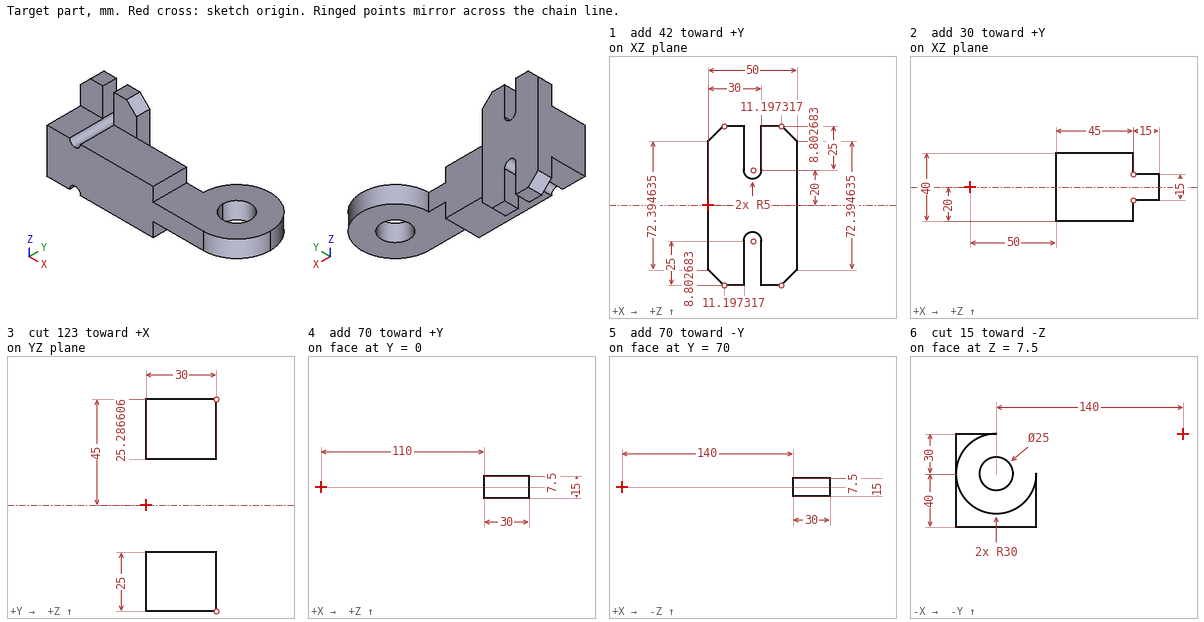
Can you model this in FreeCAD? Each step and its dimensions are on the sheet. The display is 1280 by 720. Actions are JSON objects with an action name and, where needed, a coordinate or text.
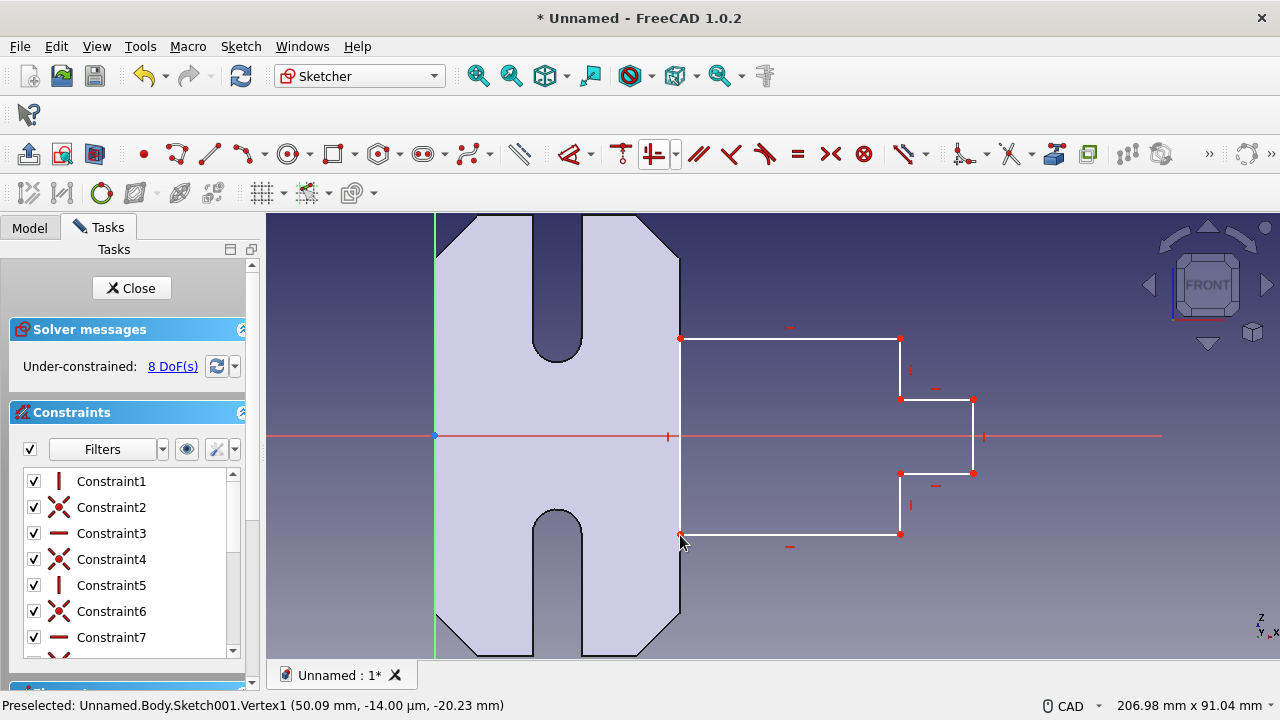
{"action": "left_click", "coordinate": [900, 400]}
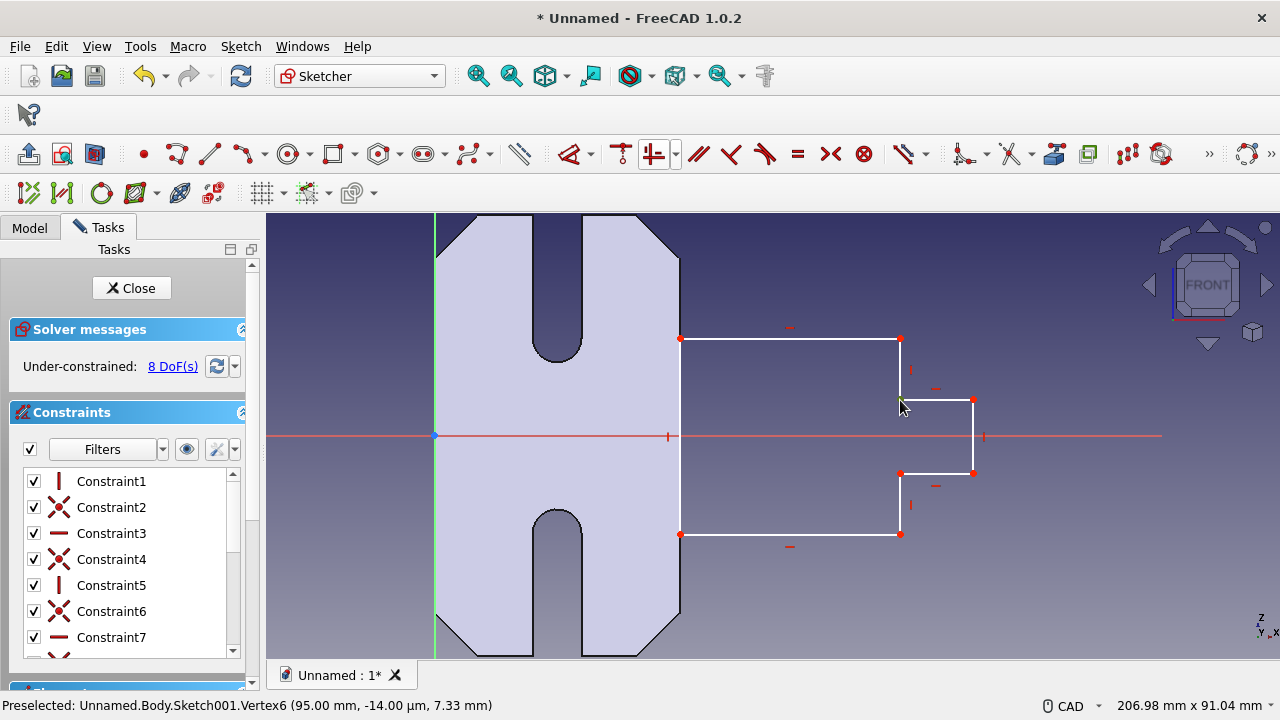
{"action": "left_click", "coordinate": [900, 474]}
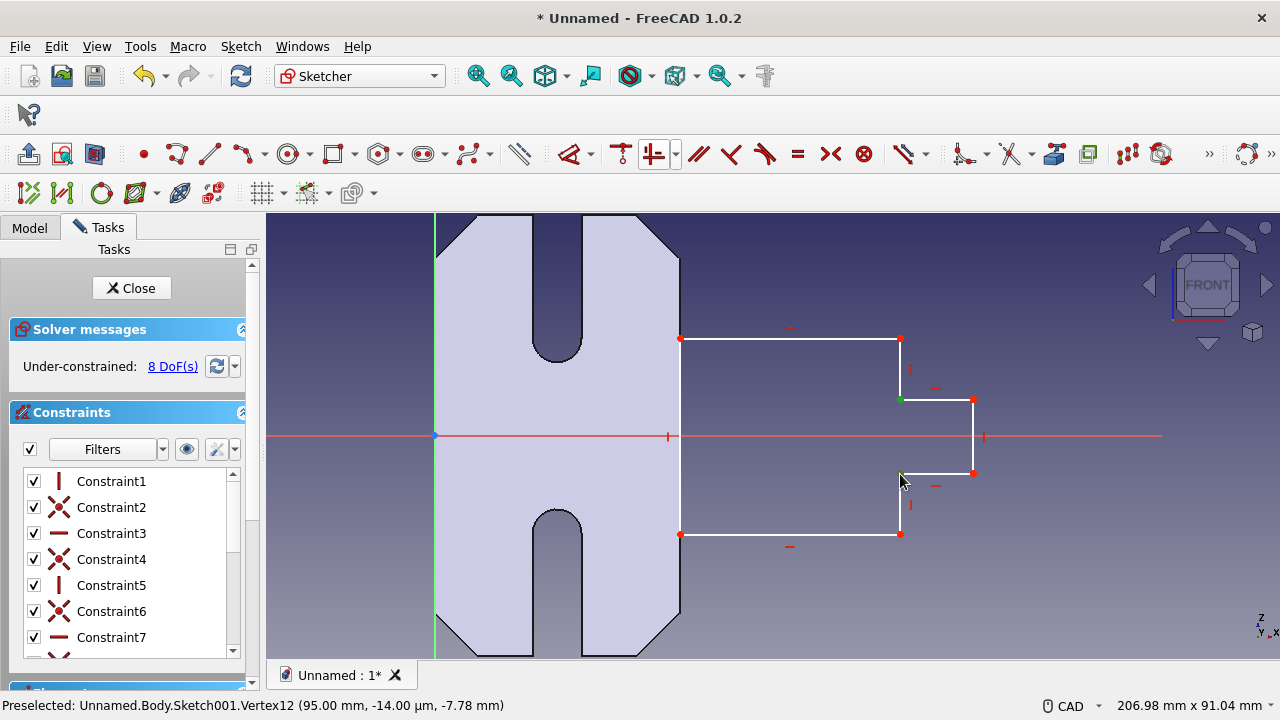
{"action": "left_click", "coordinate": [353, 436]}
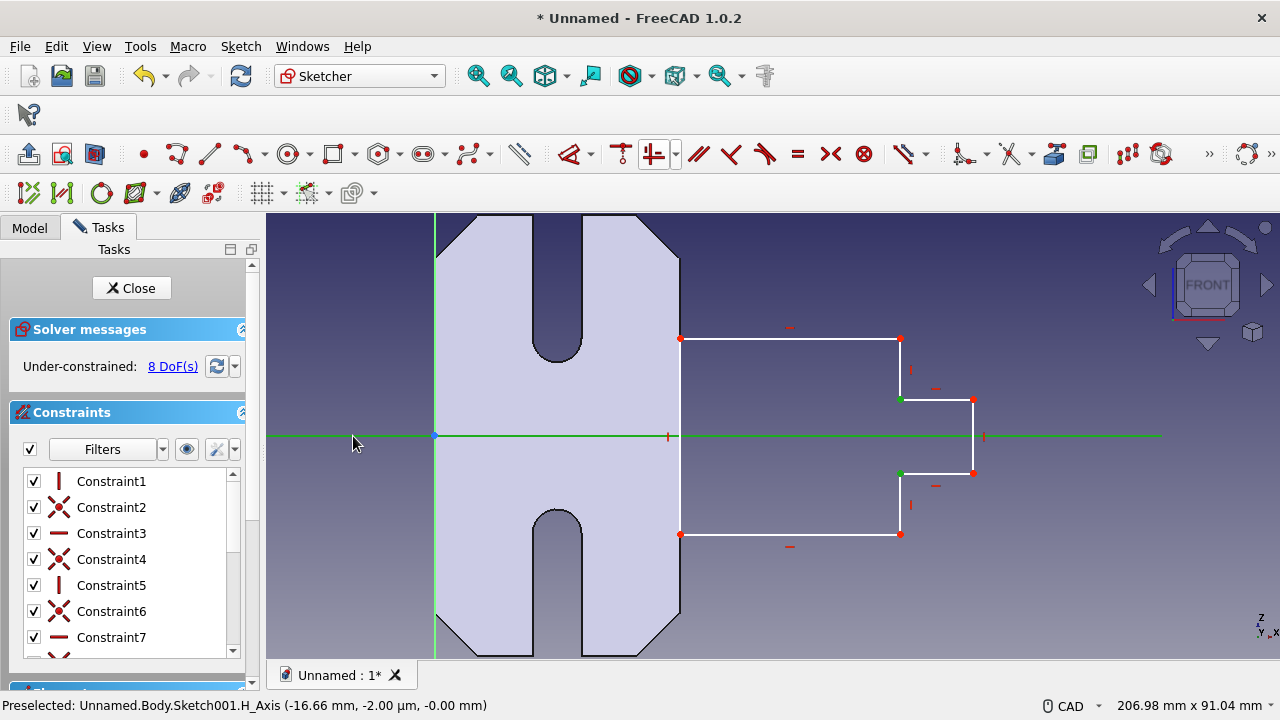
{"action": "left_click", "coordinate": [831, 154]}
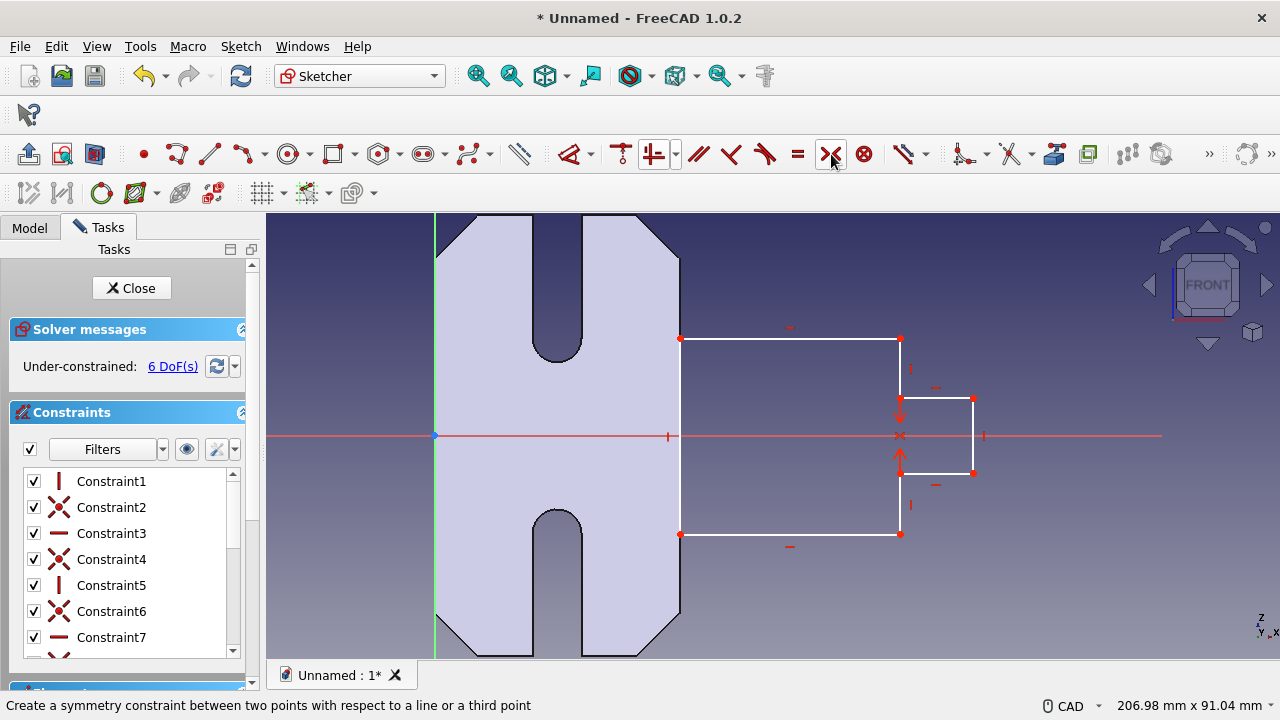
{"action": "key", "text": "d"}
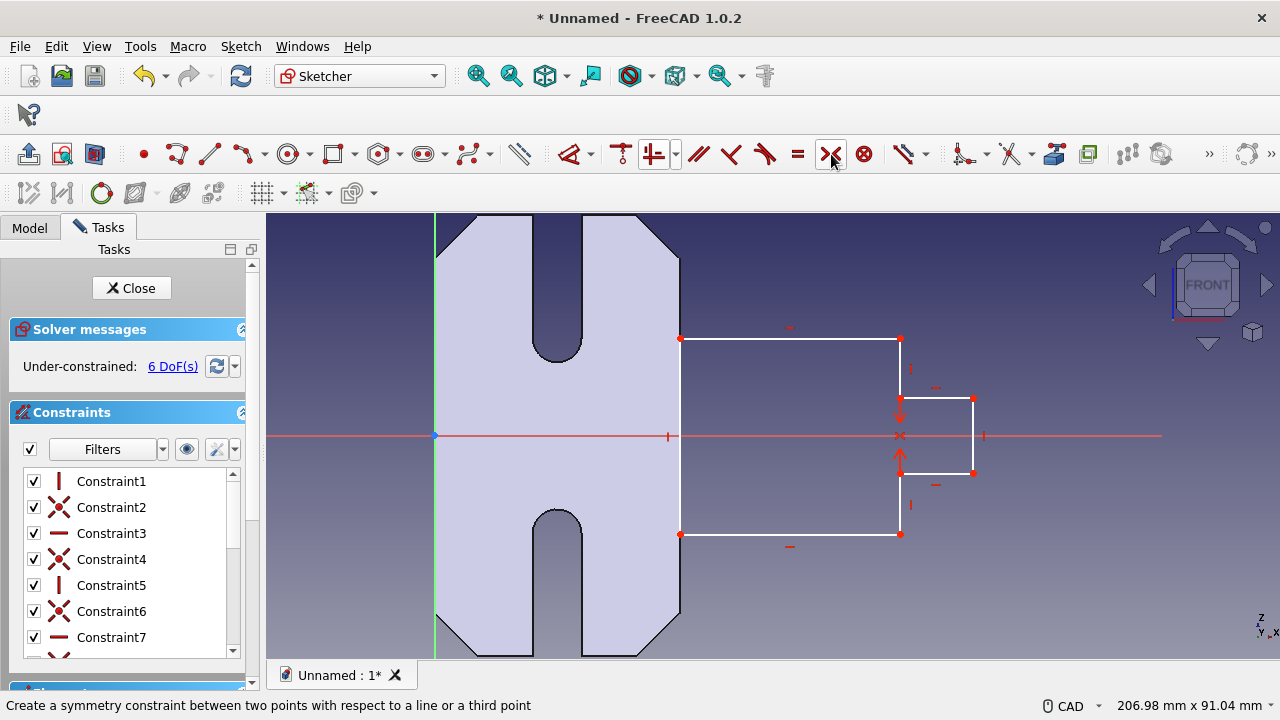
{"action": "left_click", "coordinate": [680, 476]}
{"action": "left_click", "coordinate": [646, 392]}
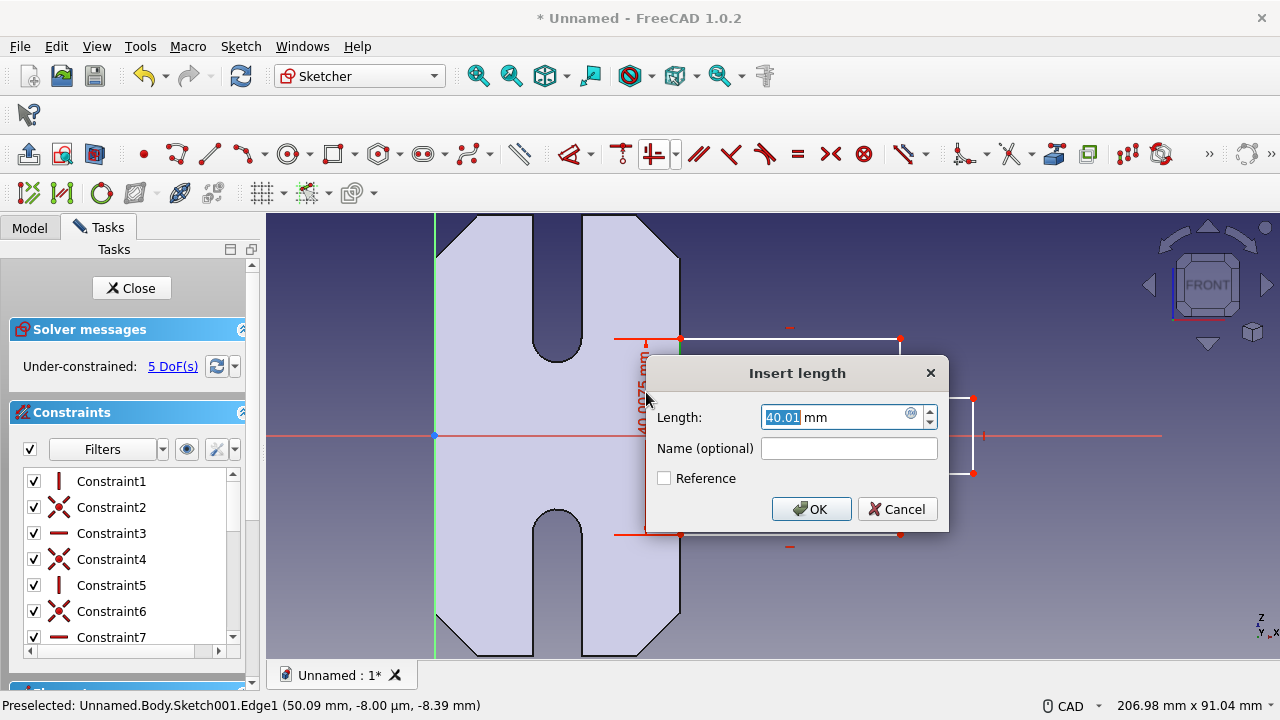
{"action": "type", "text": "40"}
{"action": "key", "text": "Return"}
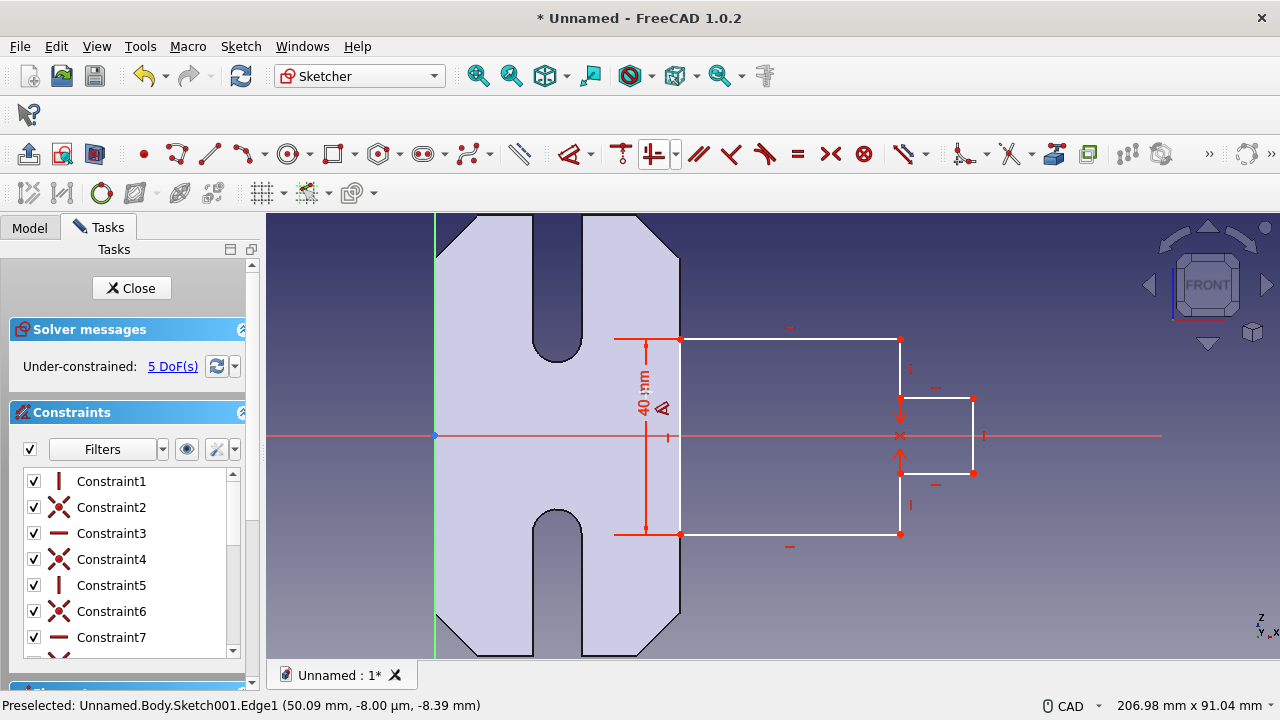
{"action": "left_click", "coordinate": [746, 339]}
{"action": "left_click", "coordinate": [790, 305]}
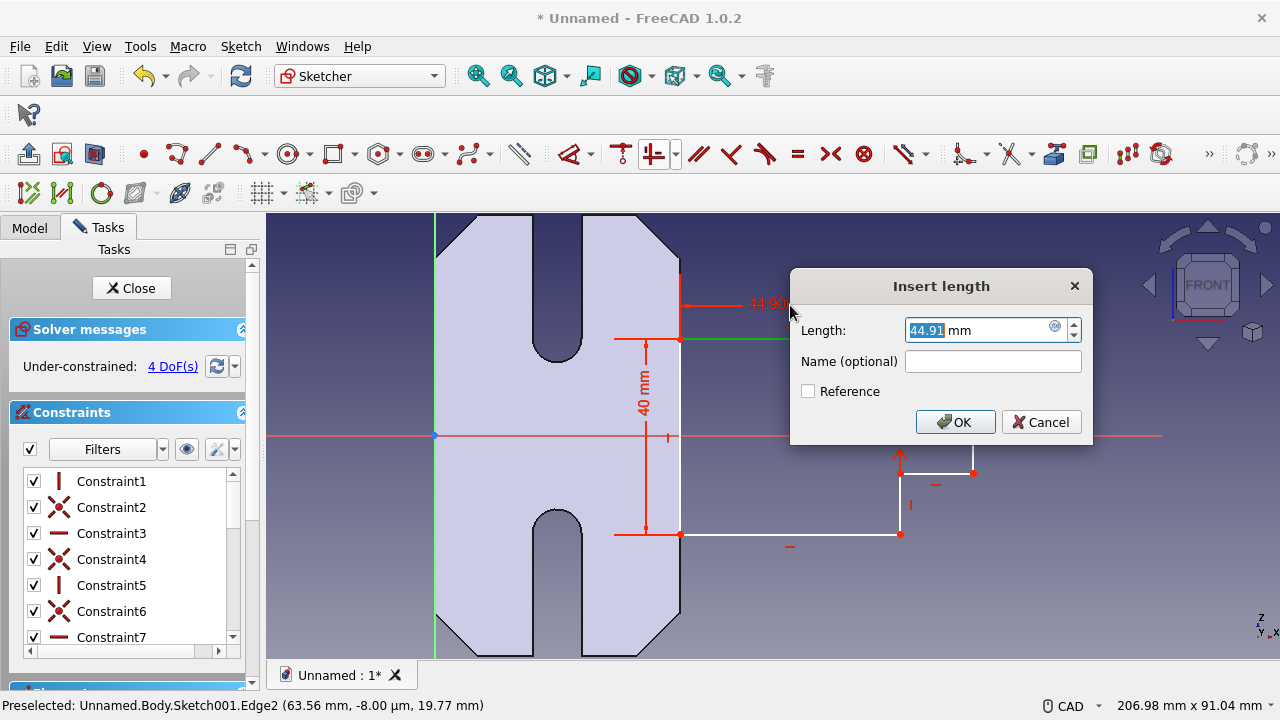
{"action": "type", "text": "45"}
{"action": "key", "text": "Return"}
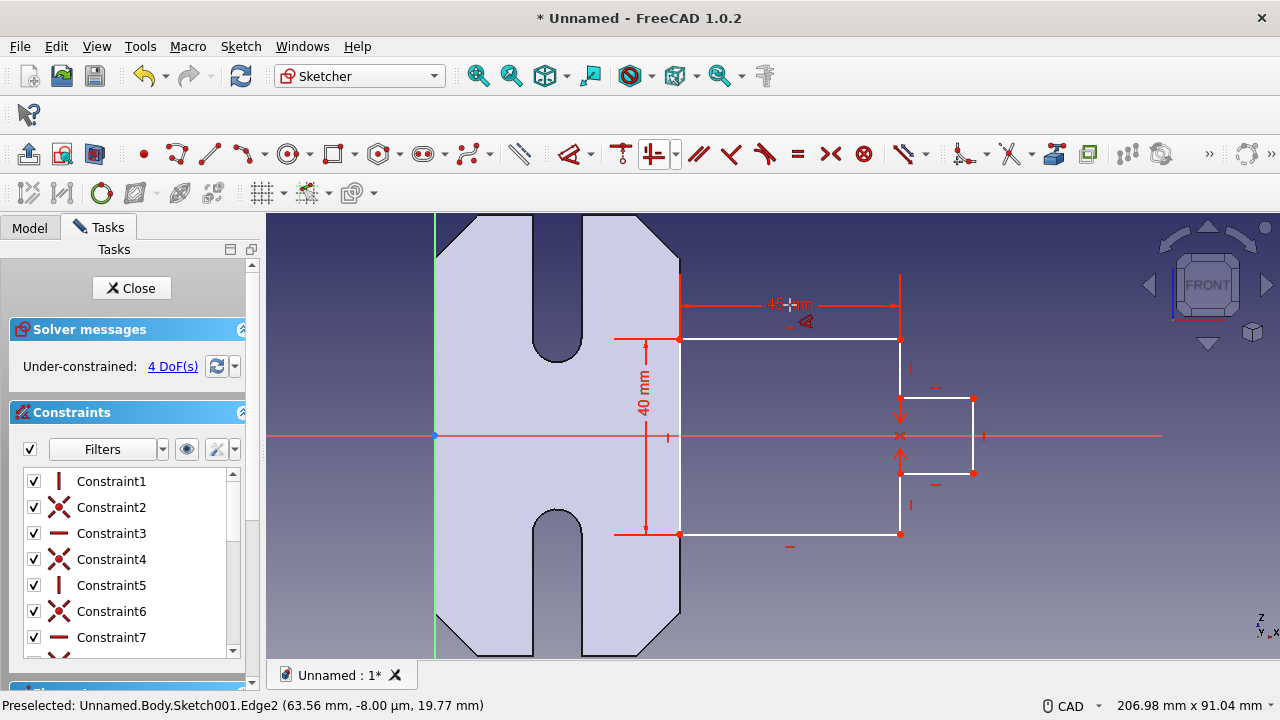
{"action": "left_click", "coordinate": [922, 398]}
{"action": "left_click", "coordinate": [937, 364]}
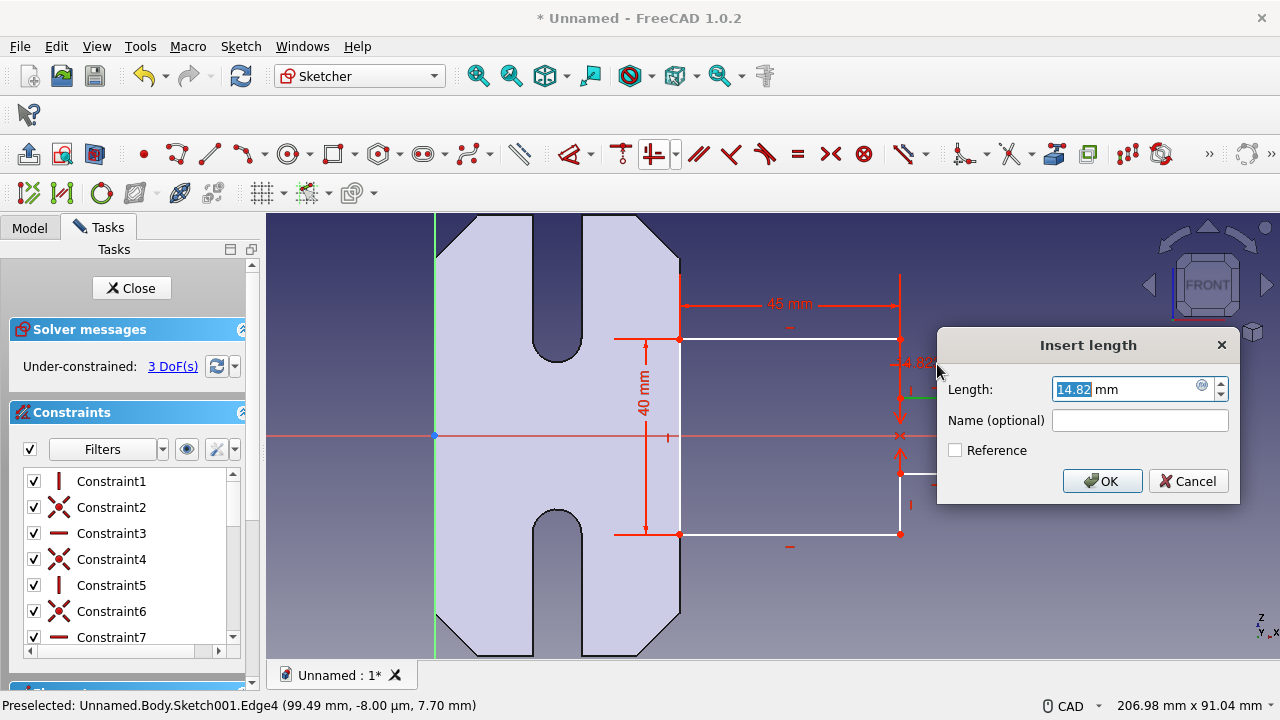
{"action": "type", "text": "15"}
{"action": "key", "text": "Return"}